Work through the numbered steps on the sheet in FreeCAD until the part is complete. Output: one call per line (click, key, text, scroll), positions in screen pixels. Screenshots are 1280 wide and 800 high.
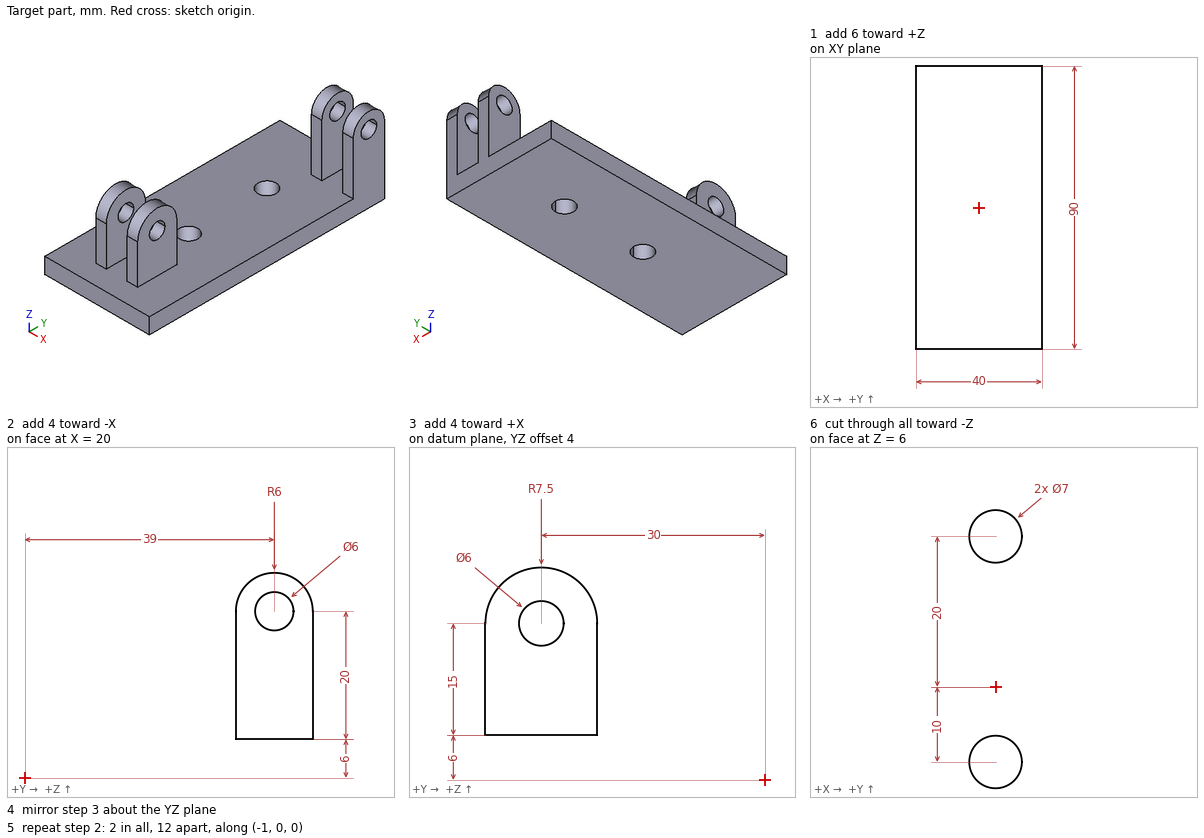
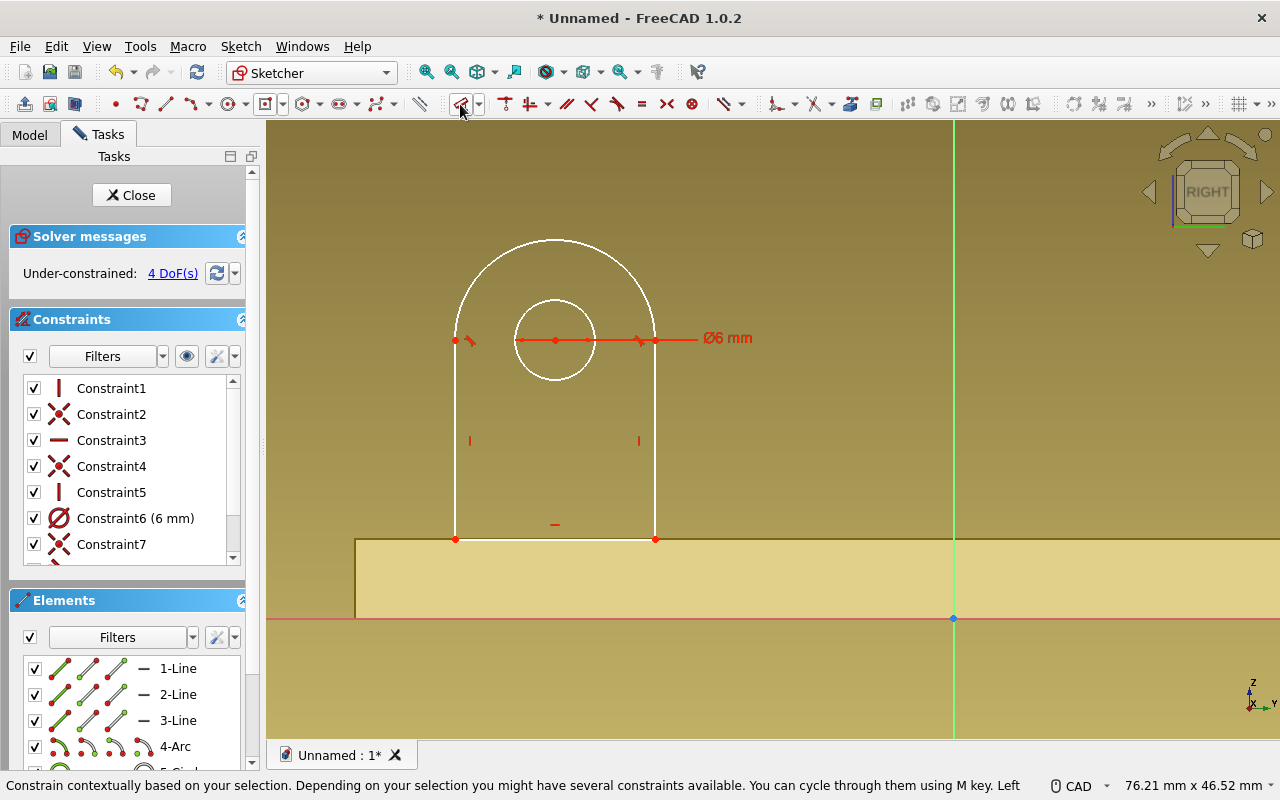
click(614, 259)
click(633, 233)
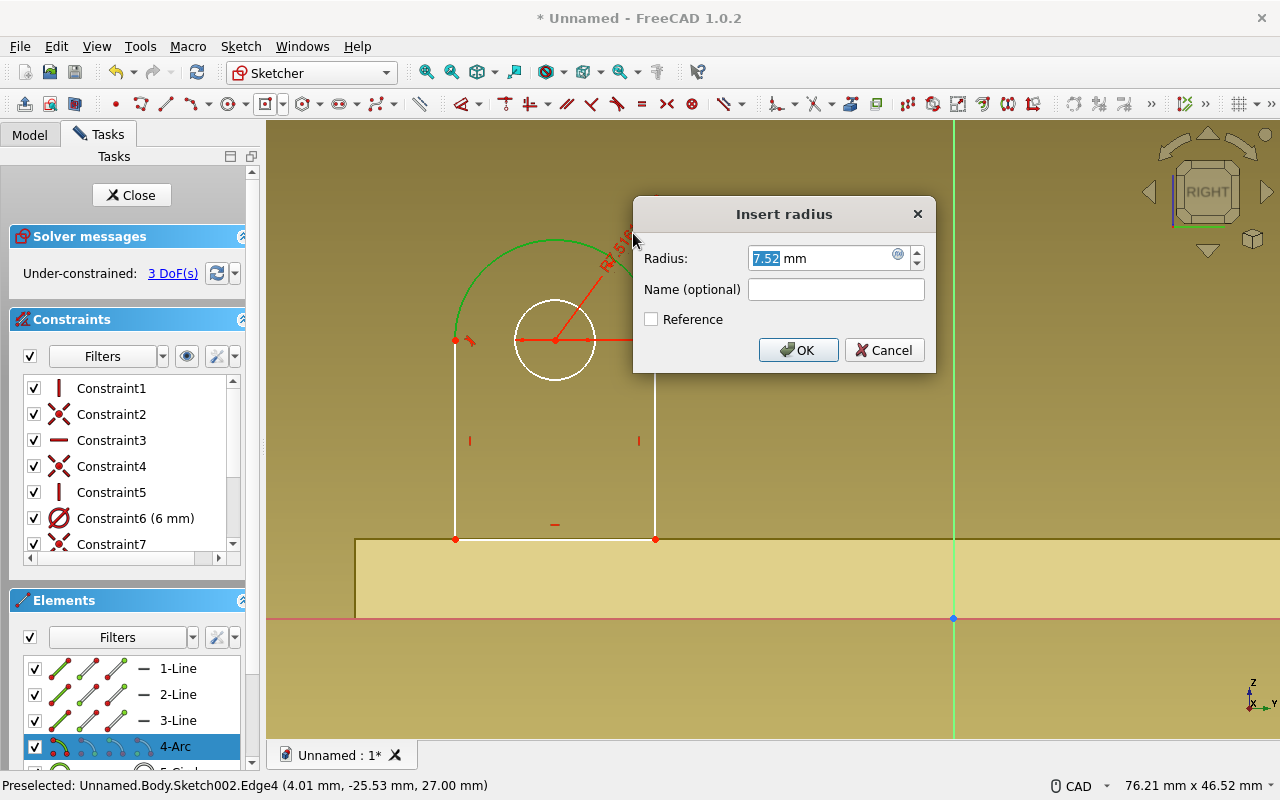
text(7.5)
key(Return)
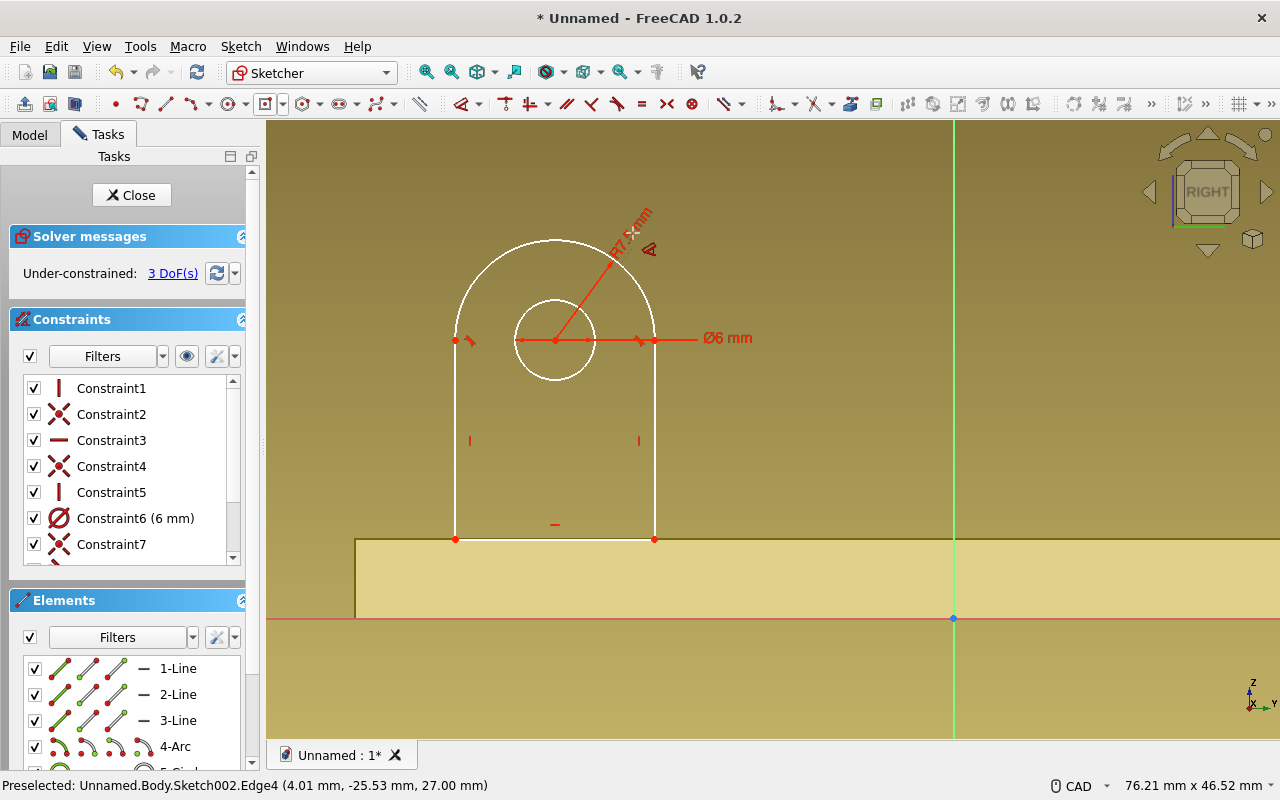
click(455, 400)
click(421, 440)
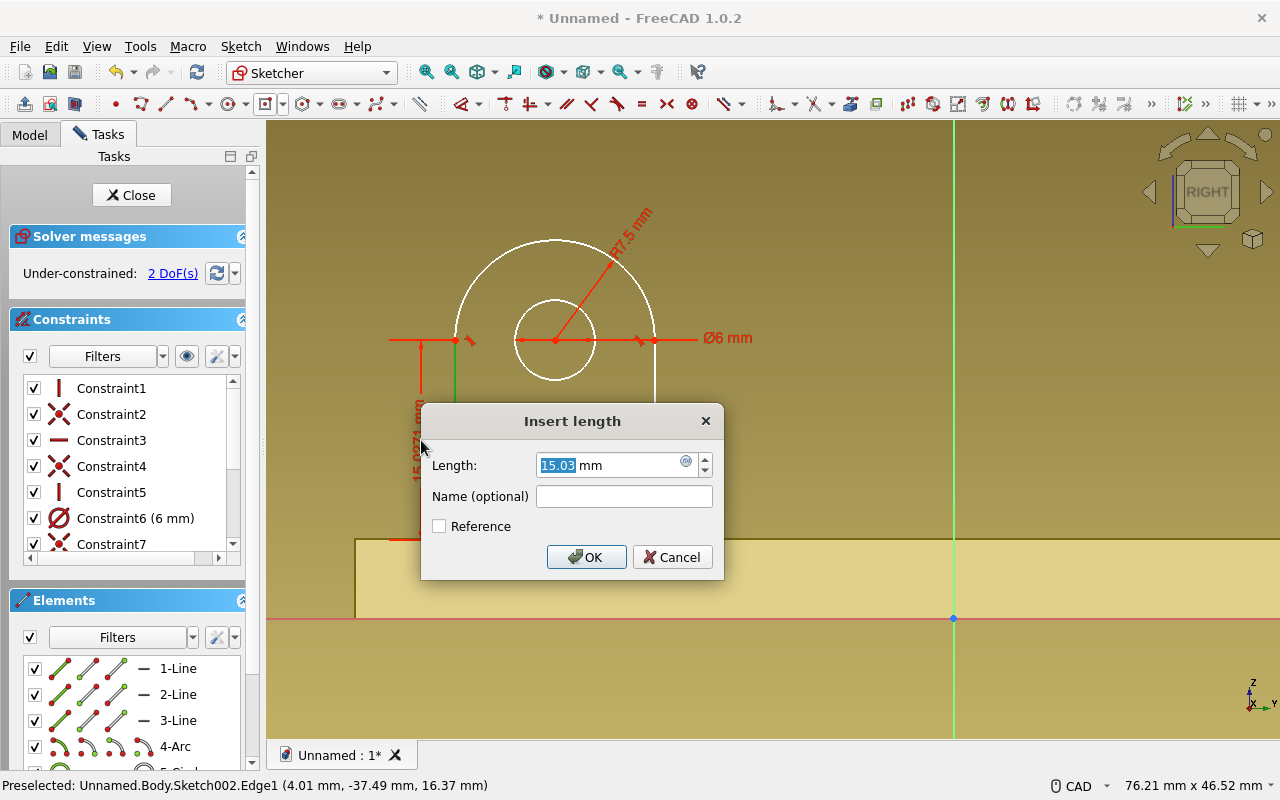
text(15)
key(Return)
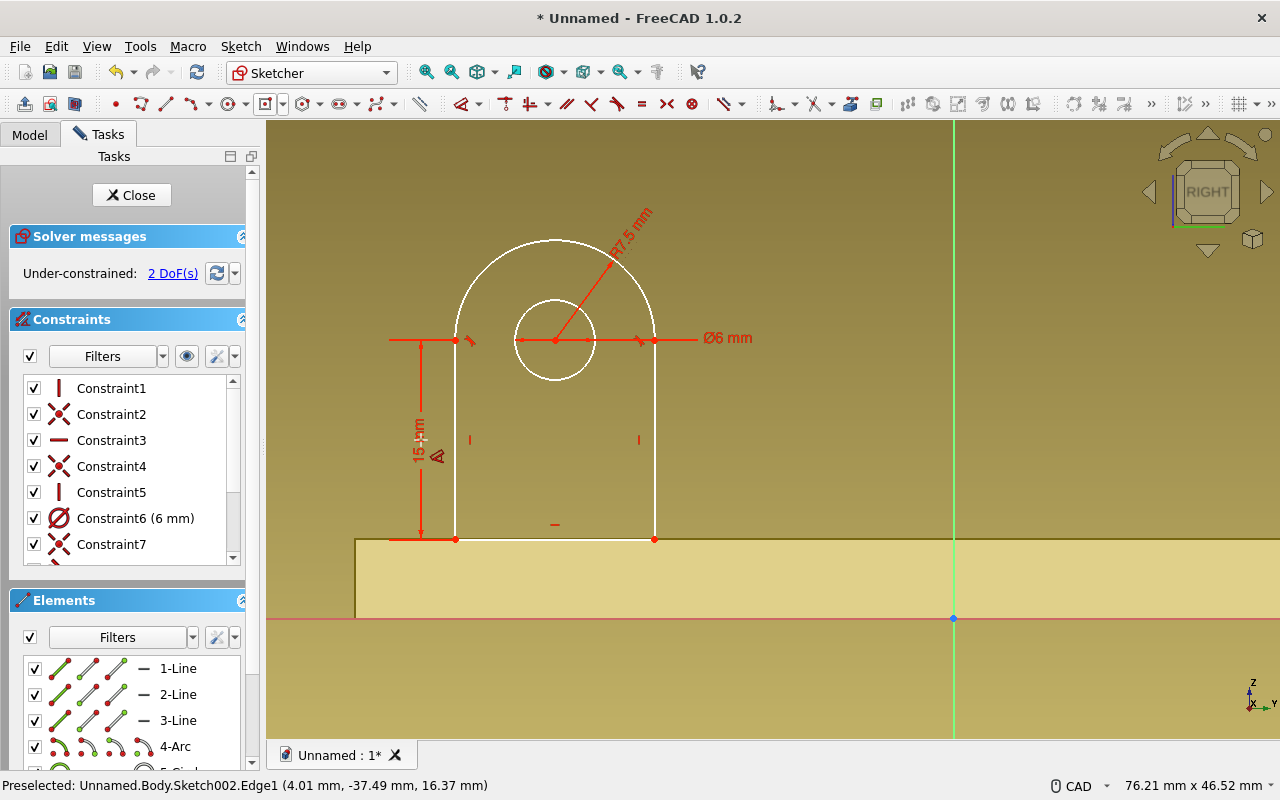
click(455, 540)
click(988, 579)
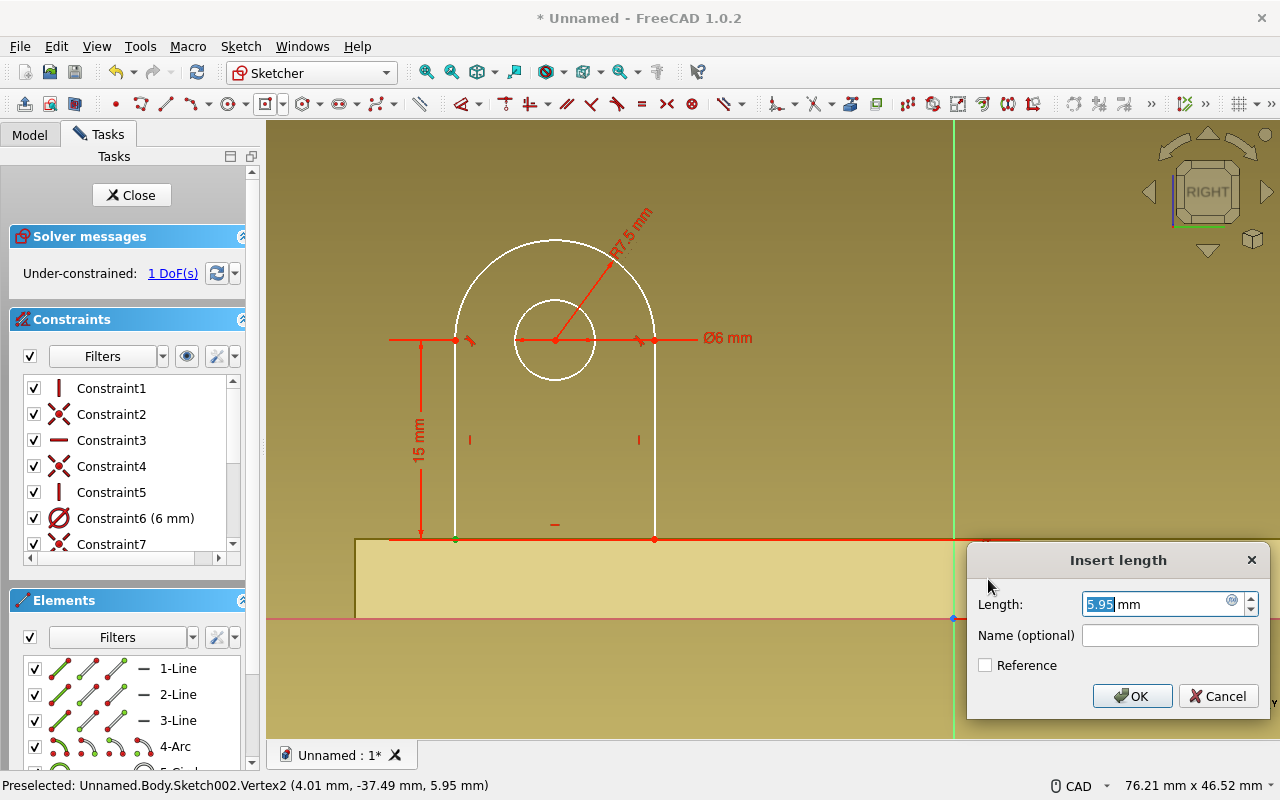
text(6)
key(Return)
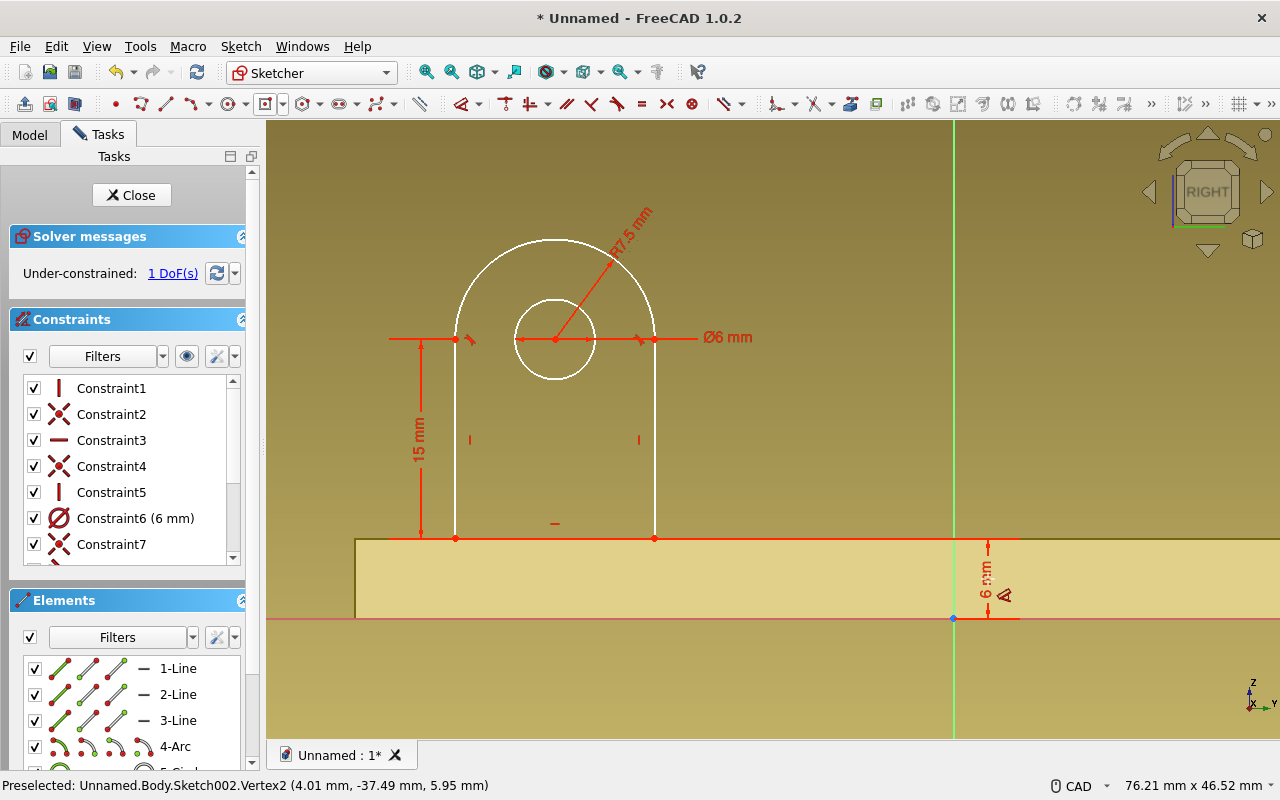
click(555, 339)
click(754, 653)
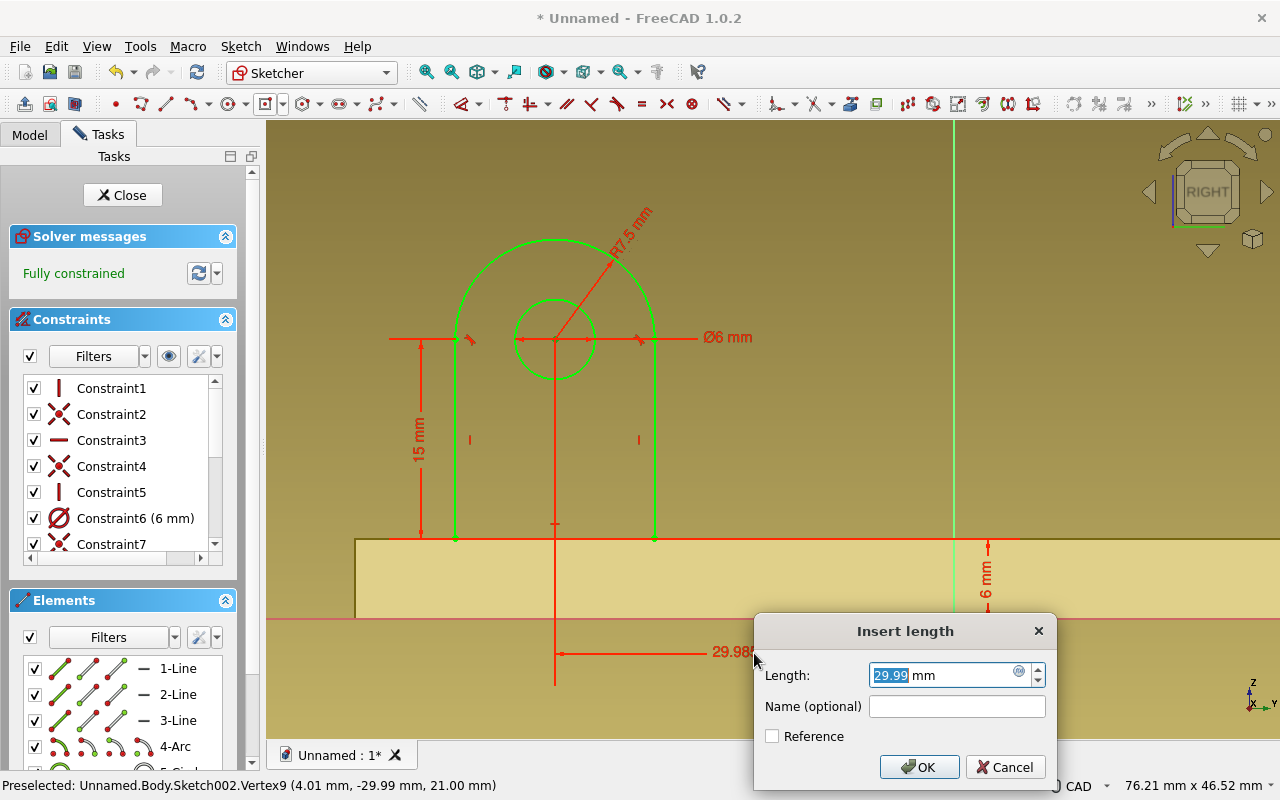
text(30)
key(Return)
key(Escape)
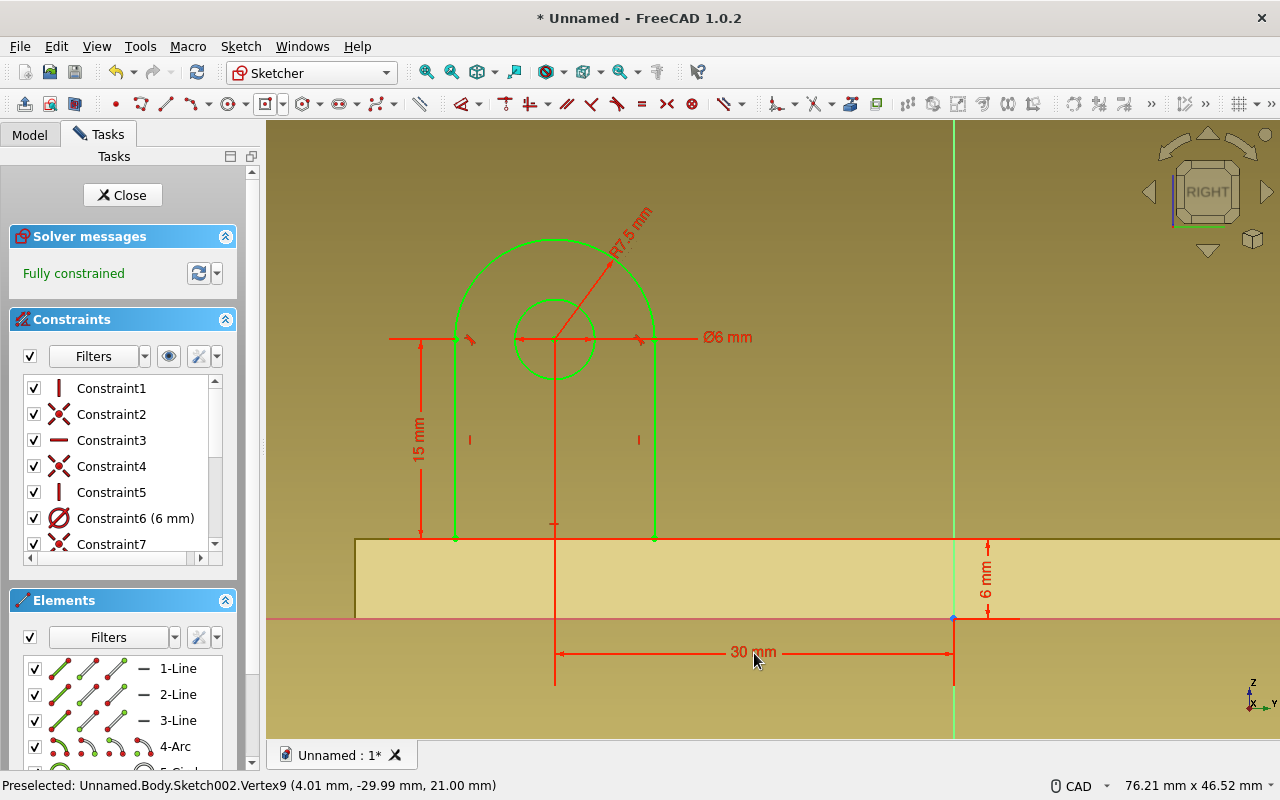
click(123, 195)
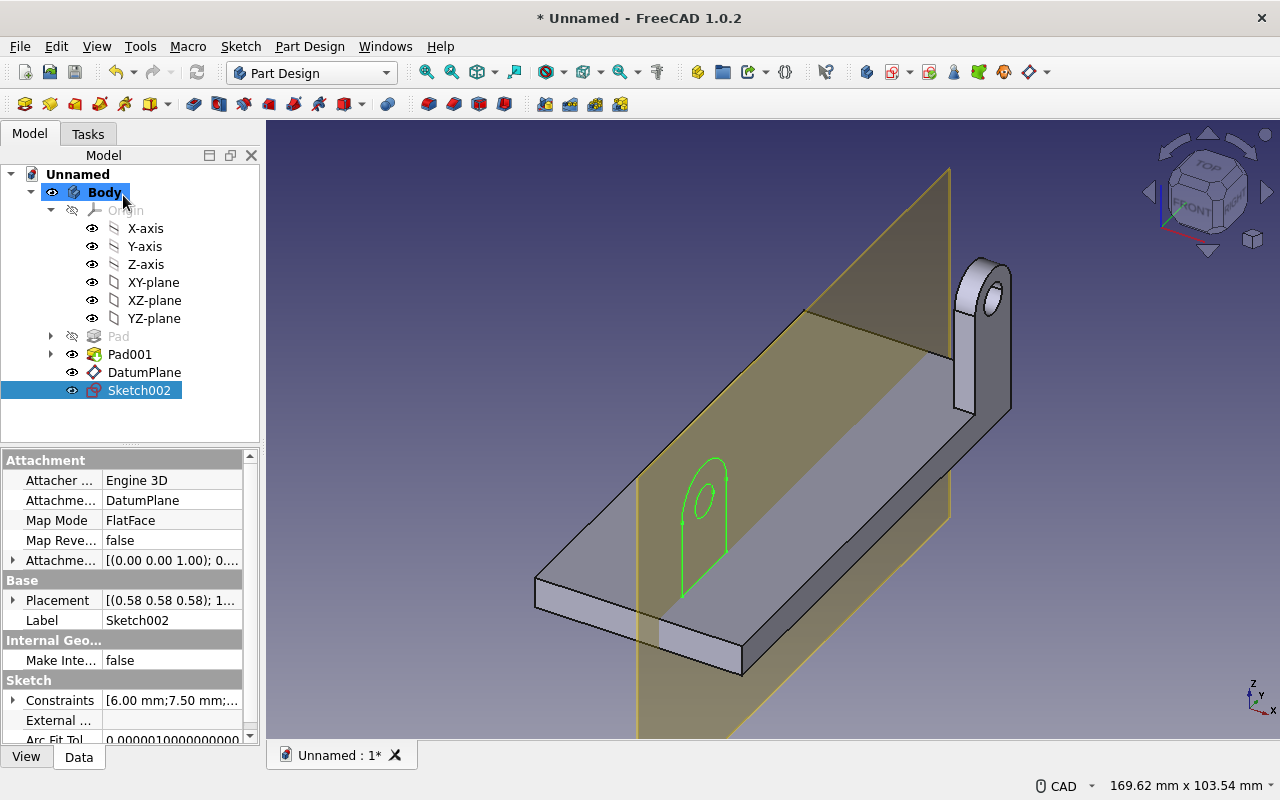
click(25, 104)